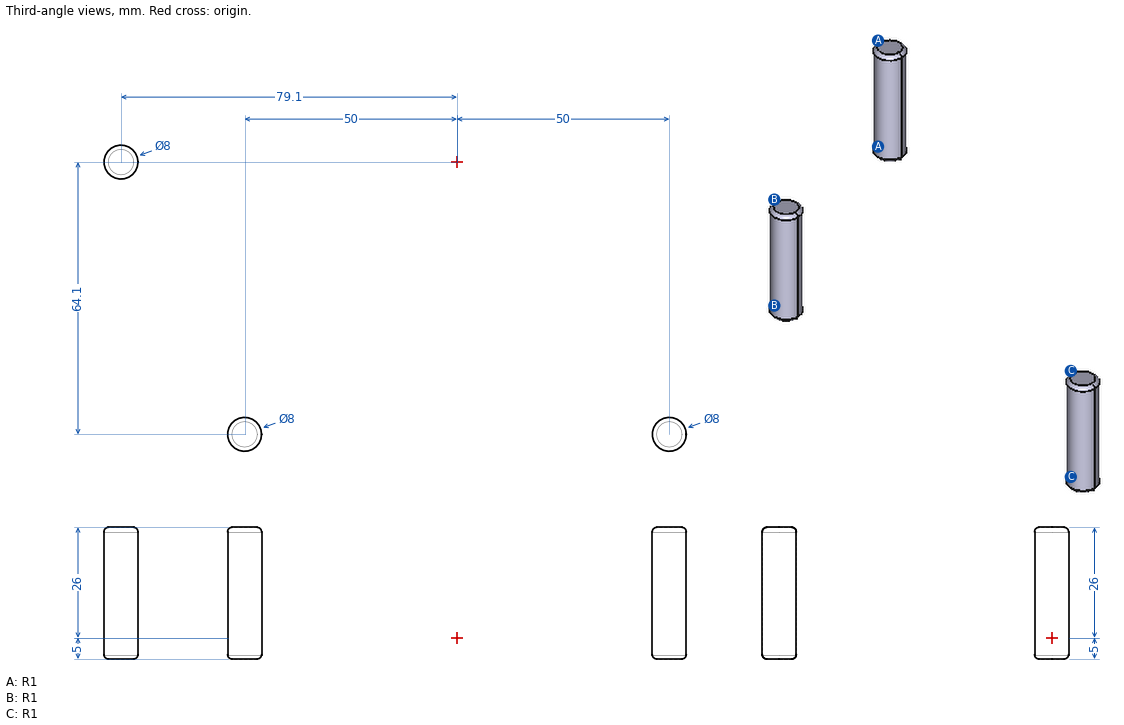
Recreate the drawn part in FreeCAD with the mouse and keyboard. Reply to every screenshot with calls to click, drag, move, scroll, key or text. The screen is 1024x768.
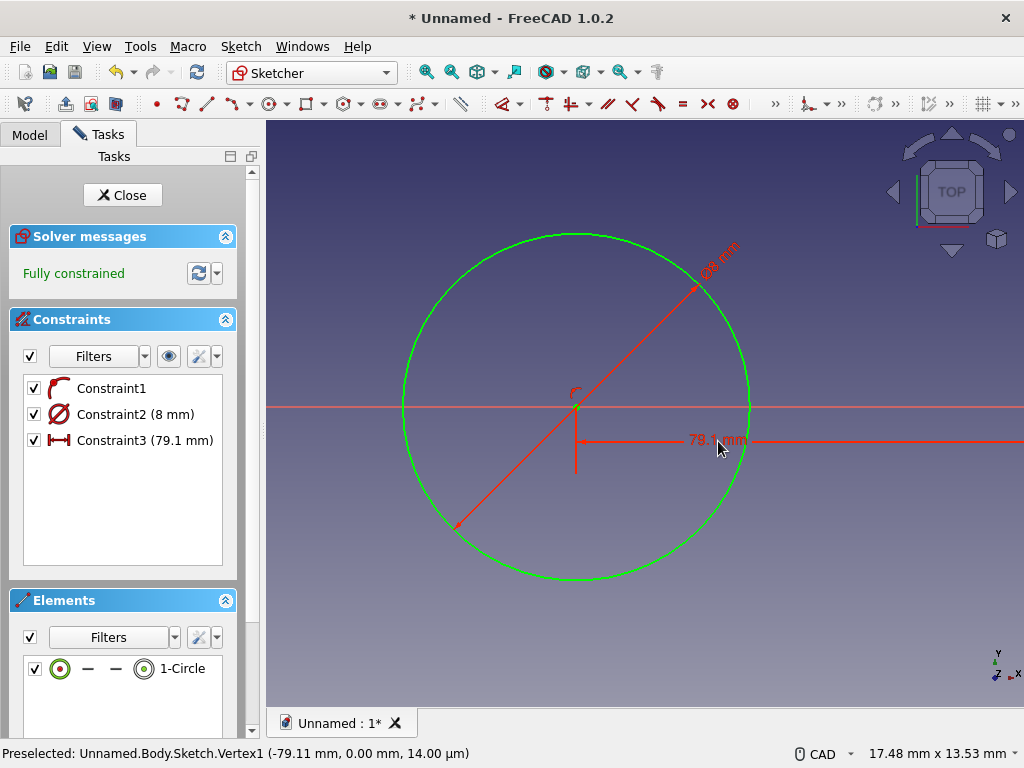
click(123, 195)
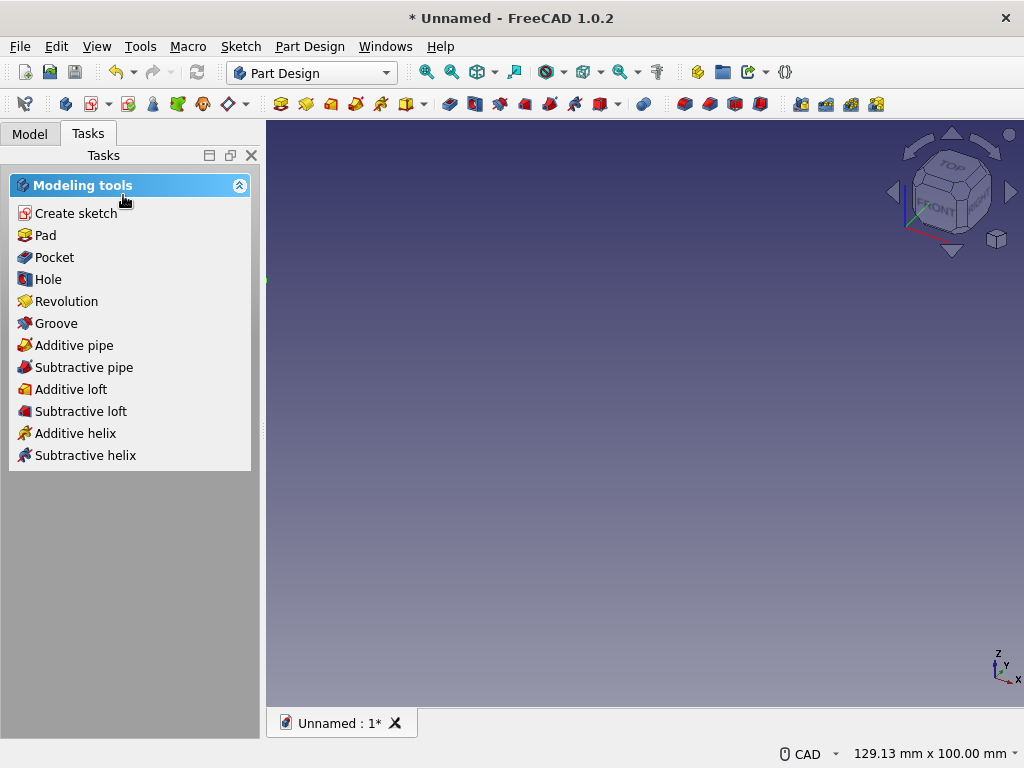
click(281, 104)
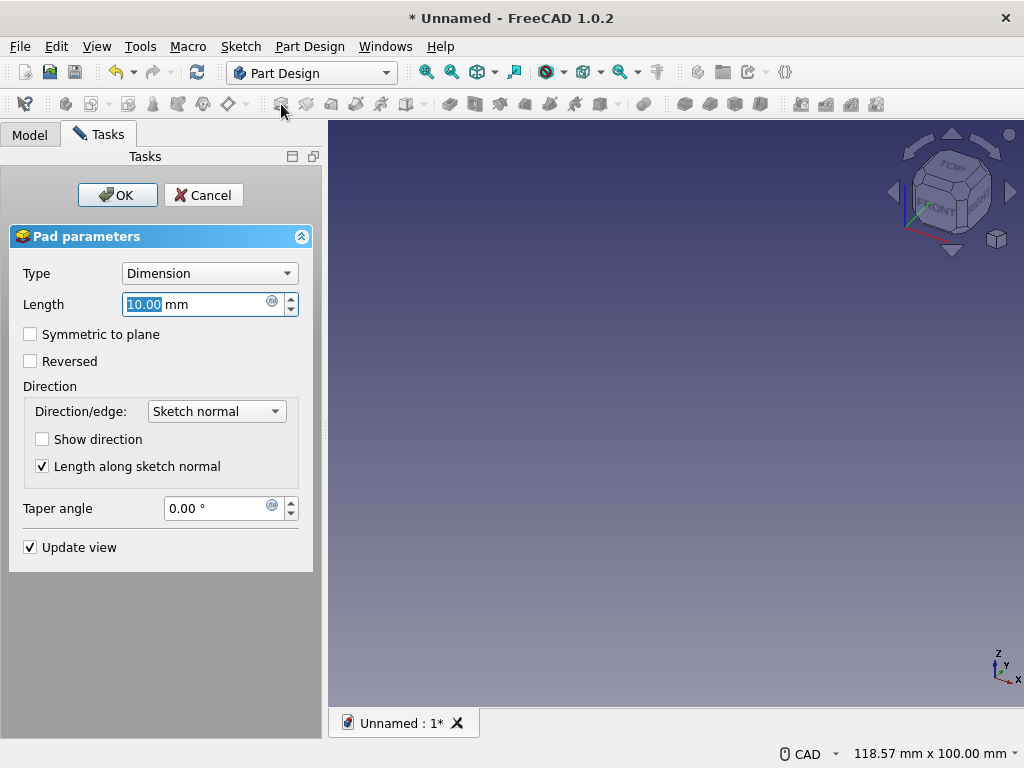
click(210, 274)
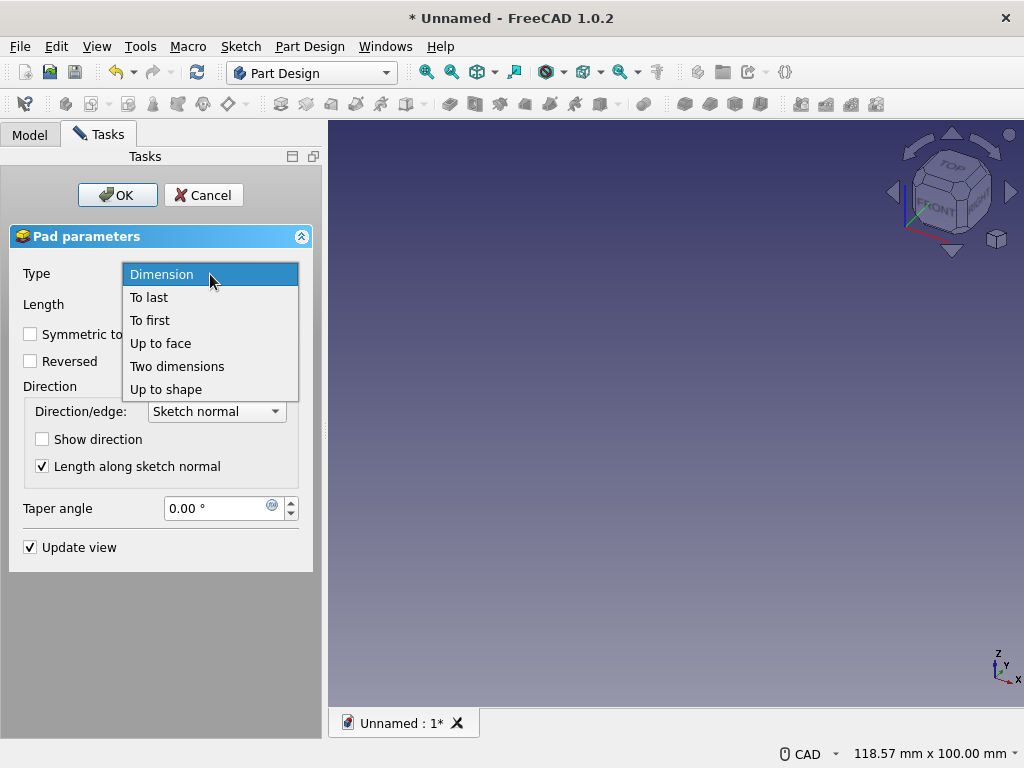
click(208, 366)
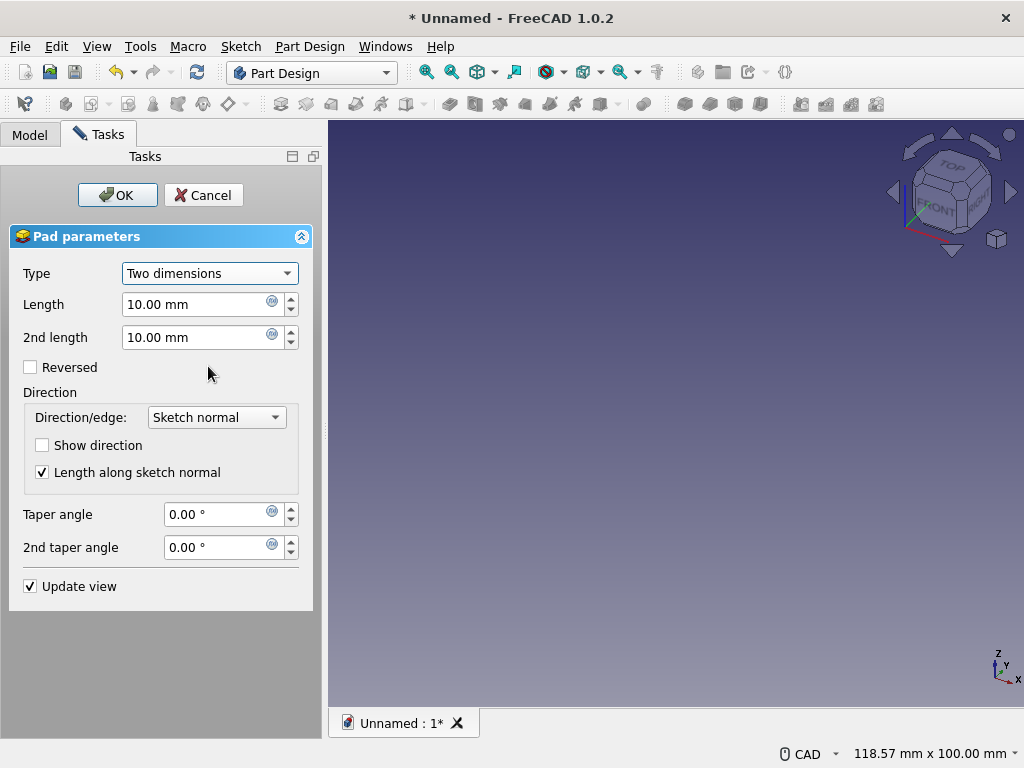
triple_click(204, 304)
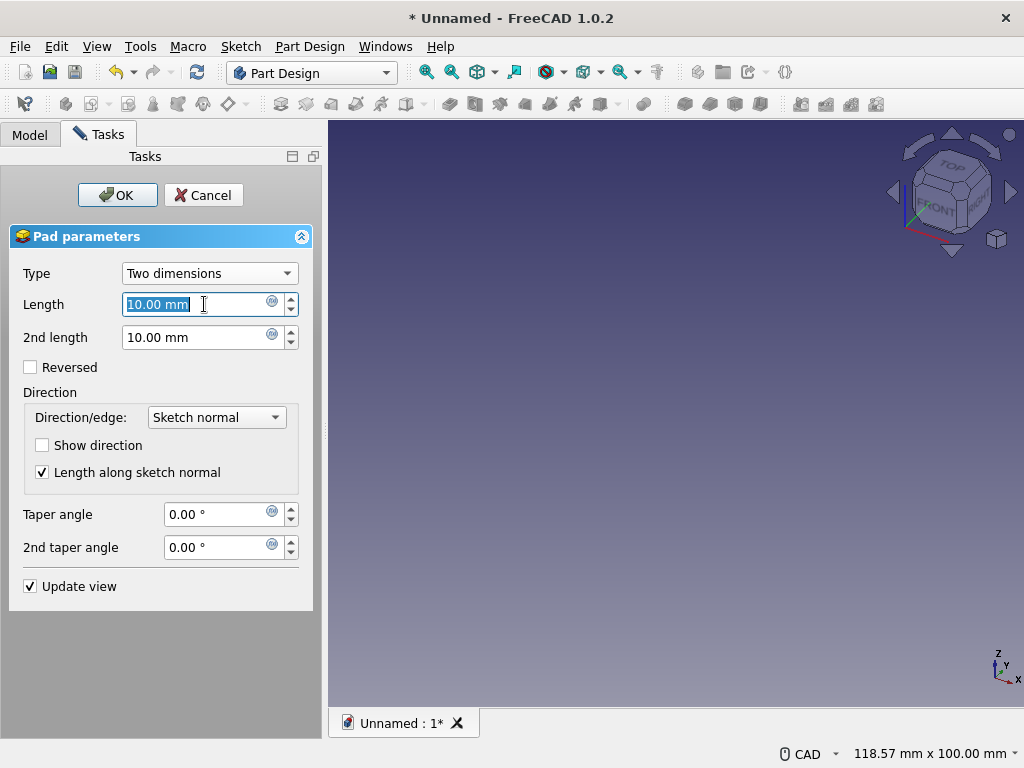
text(26)
key(Tab)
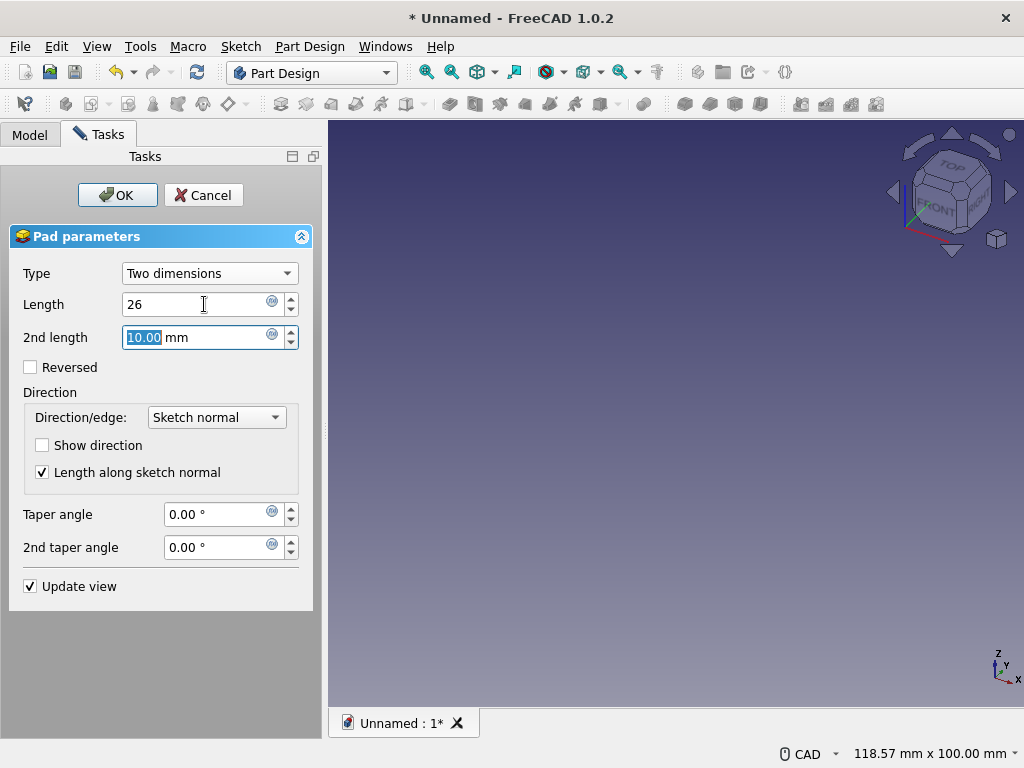
text(5)
key(Tab)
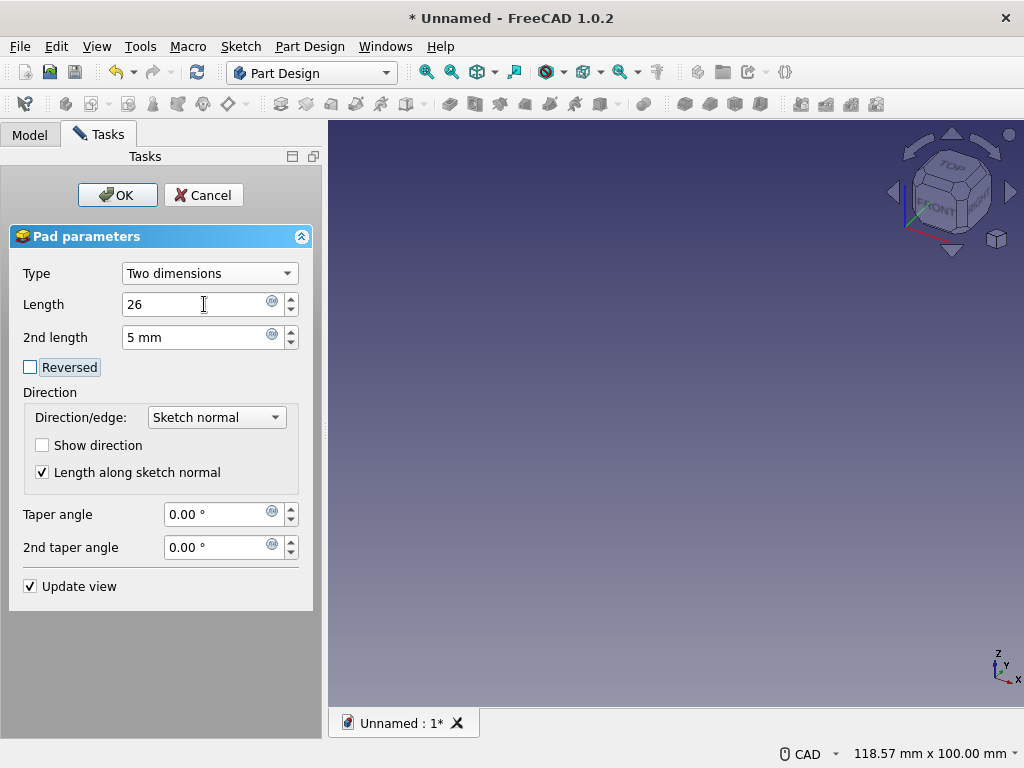
click(118, 195)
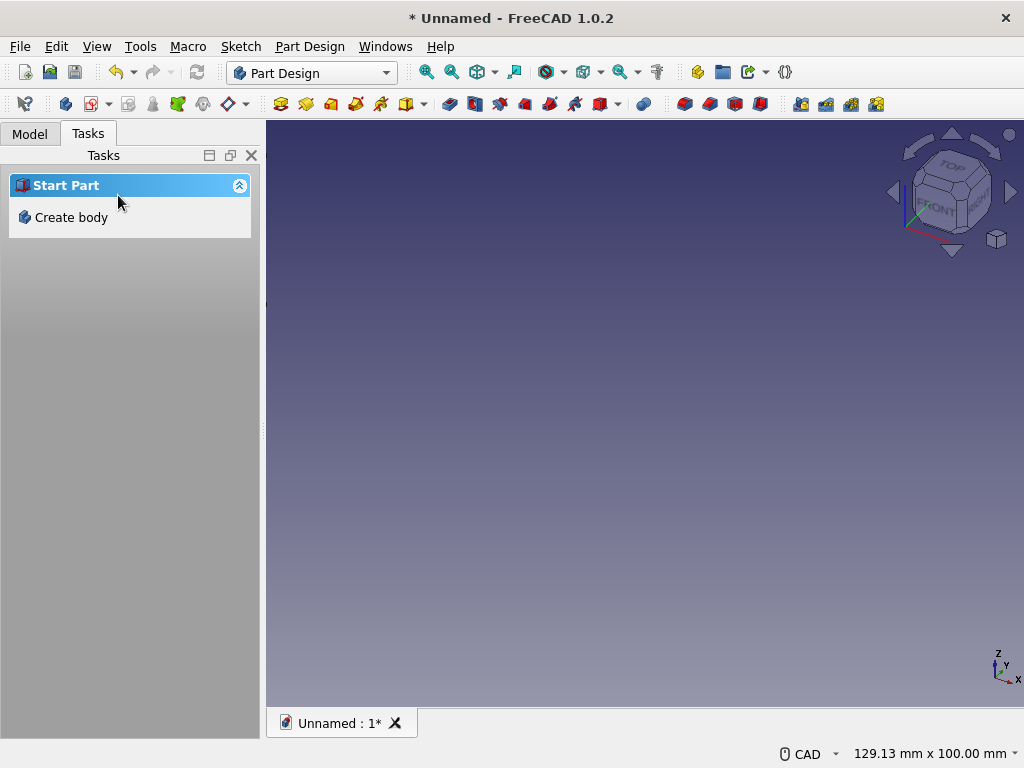
click(427, 72)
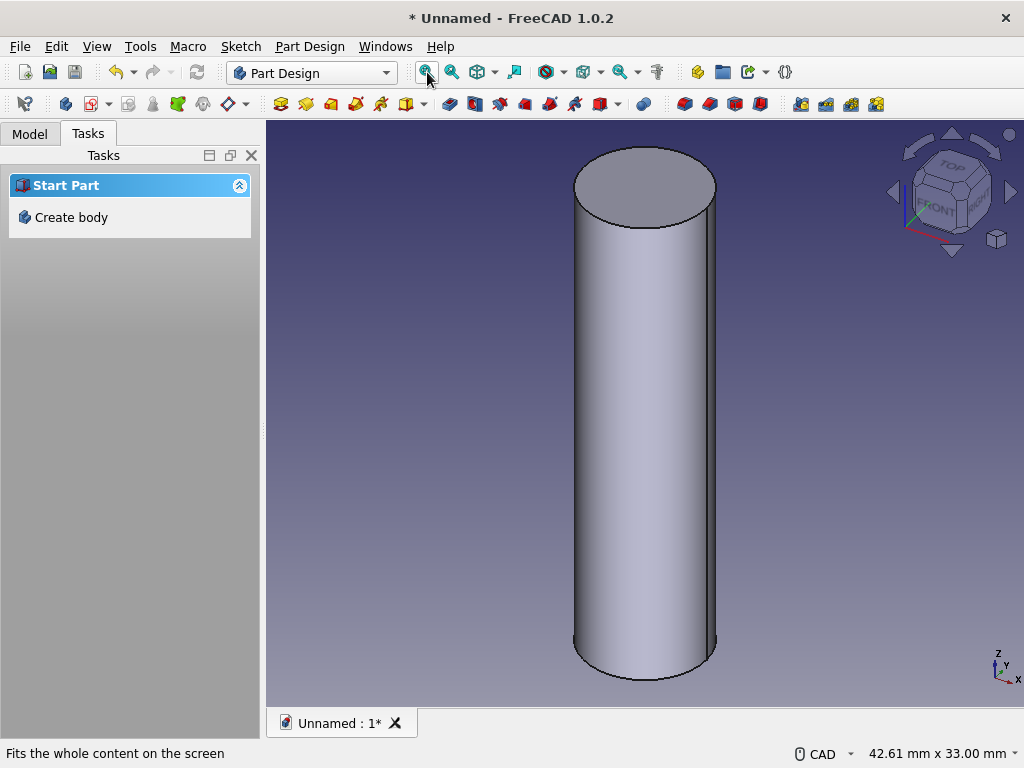
click(574, 191)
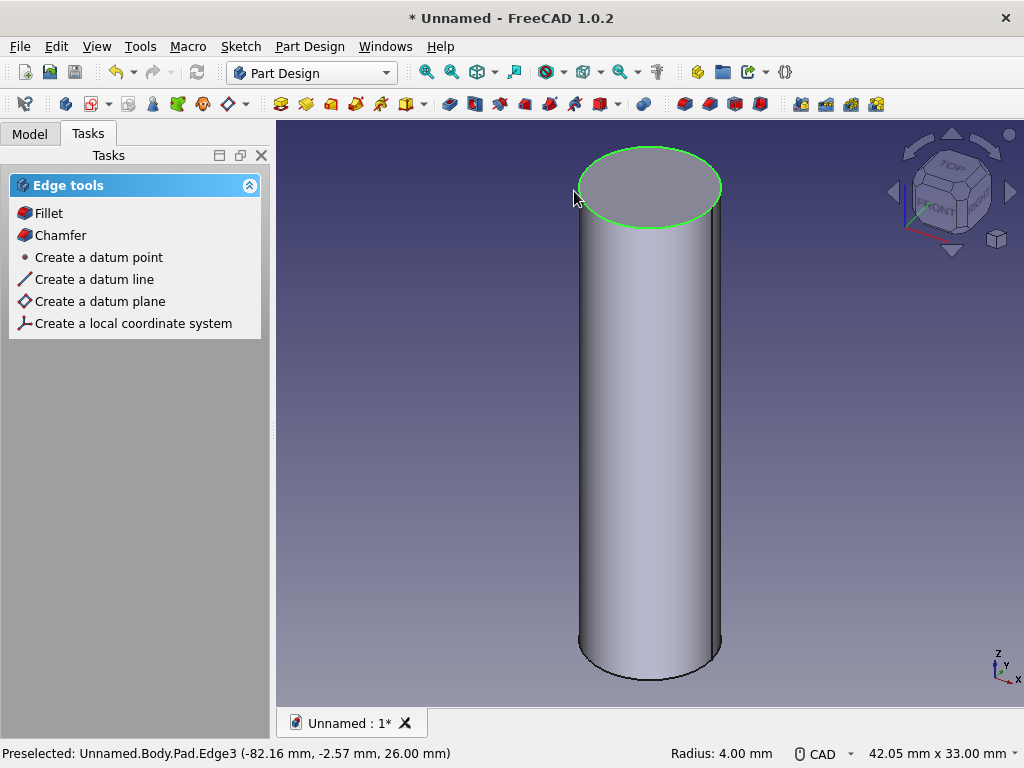
key(0)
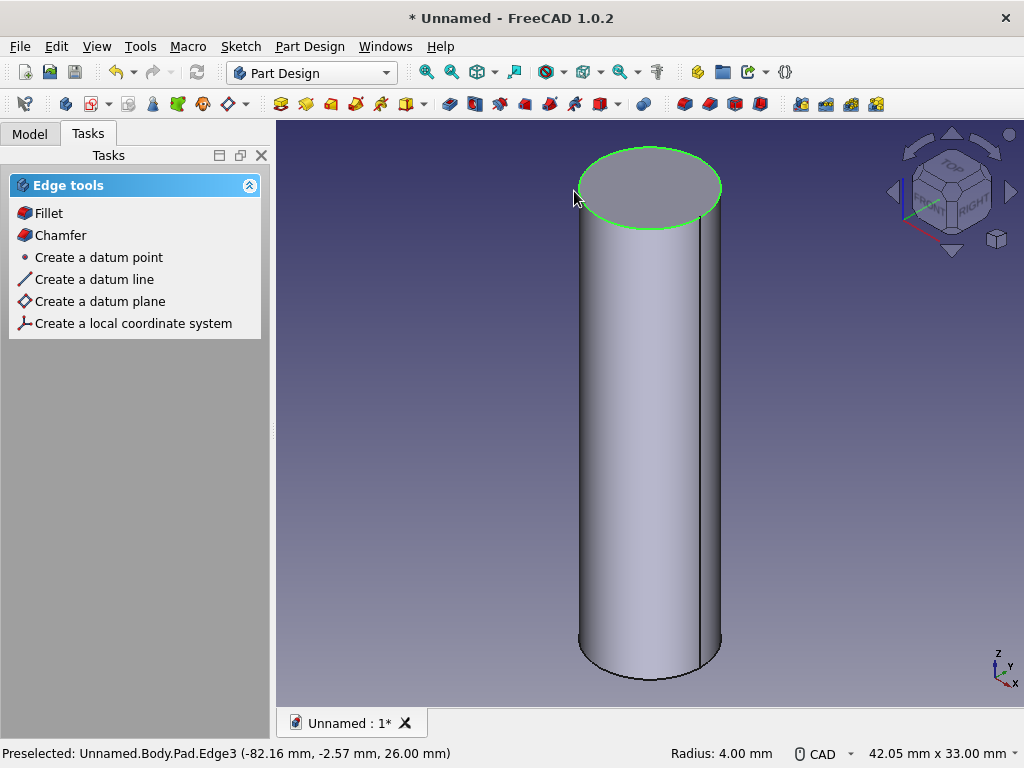
key(2)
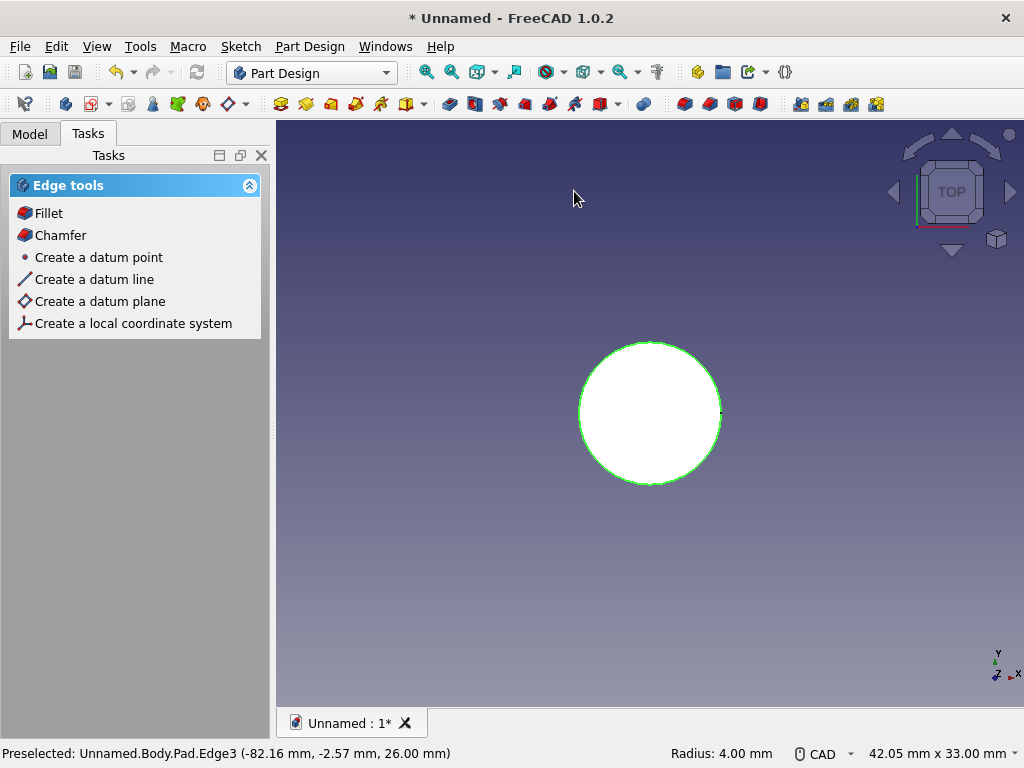
click(427, 72)